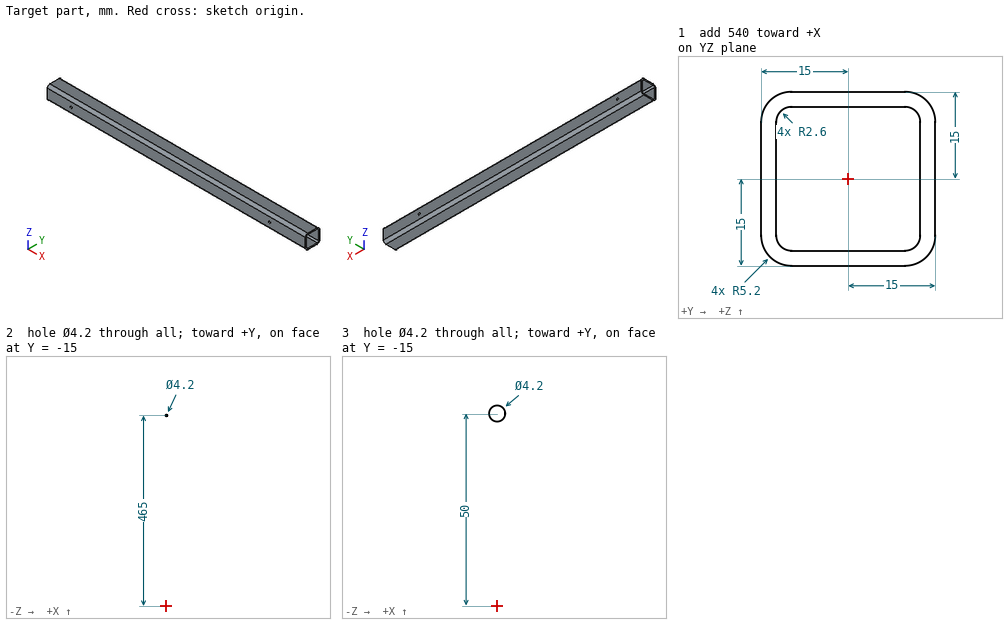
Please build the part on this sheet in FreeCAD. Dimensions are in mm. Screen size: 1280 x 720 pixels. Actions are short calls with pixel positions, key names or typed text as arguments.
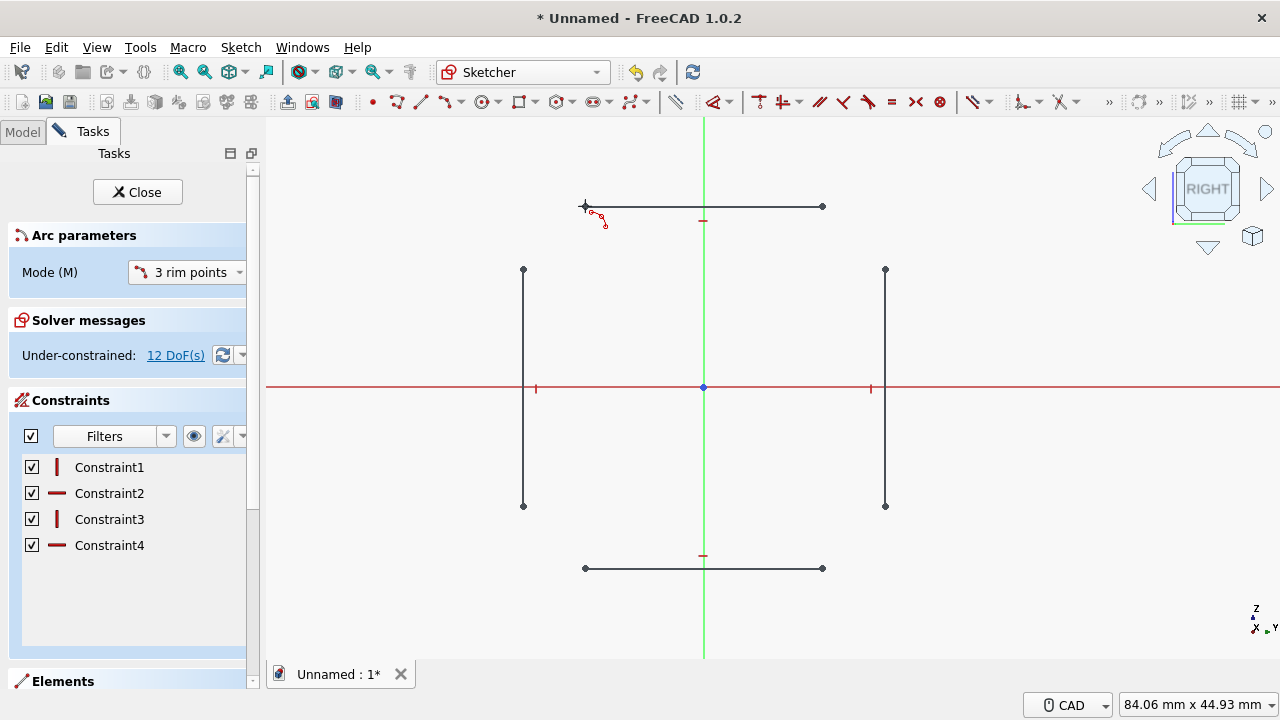
click(523, 507)
click(585, 569)
click(541, 550)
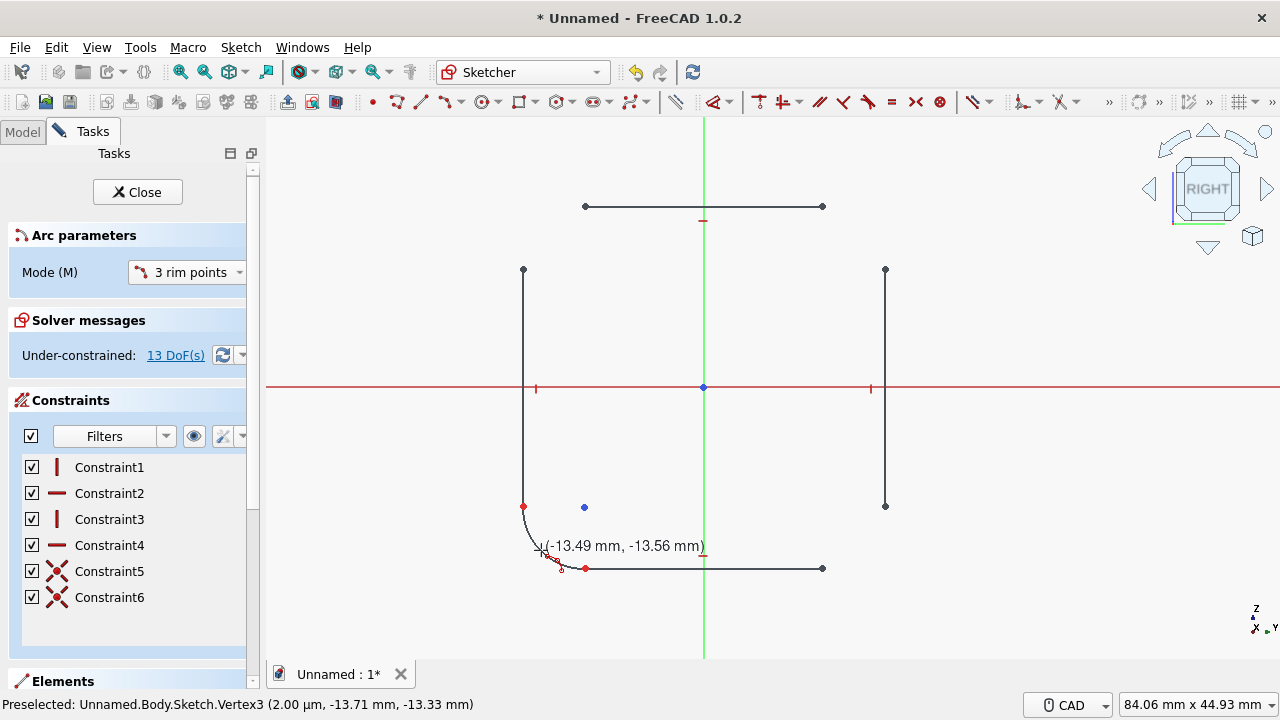
click(822, 569)
click(885, 507)
click(866, 550)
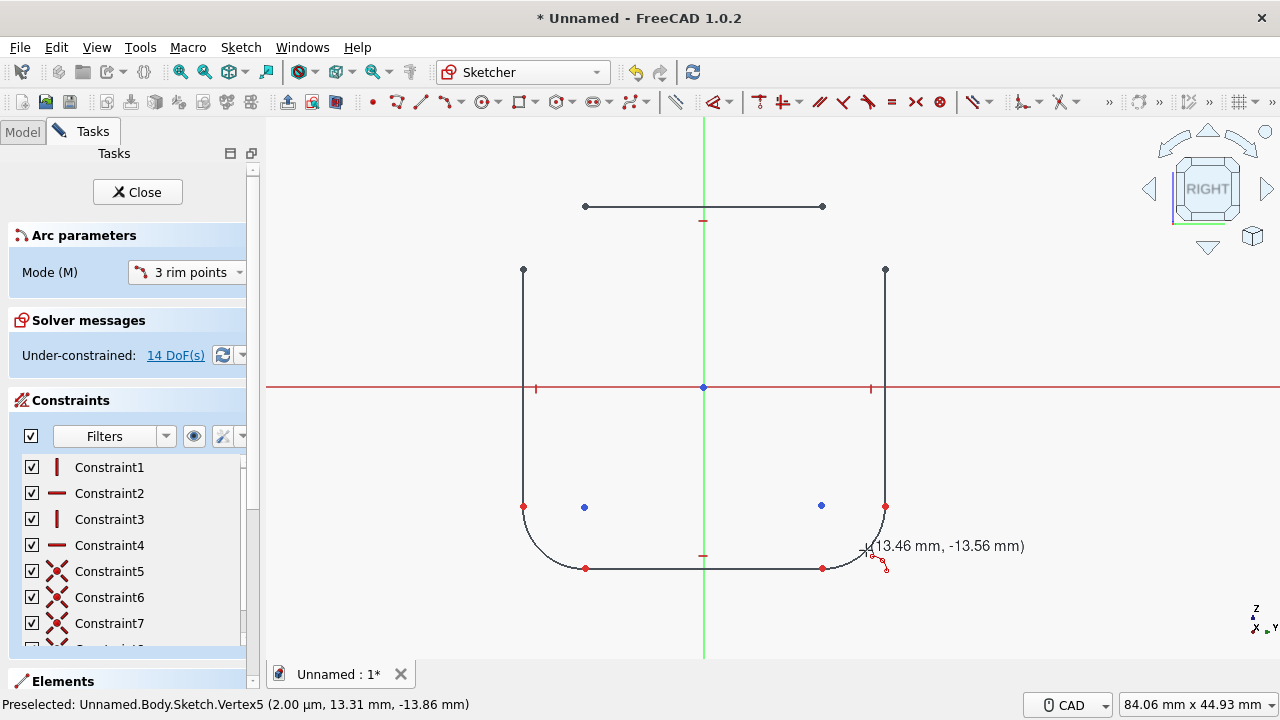
click(885, 270)
click(822, 207)
click(866, 225)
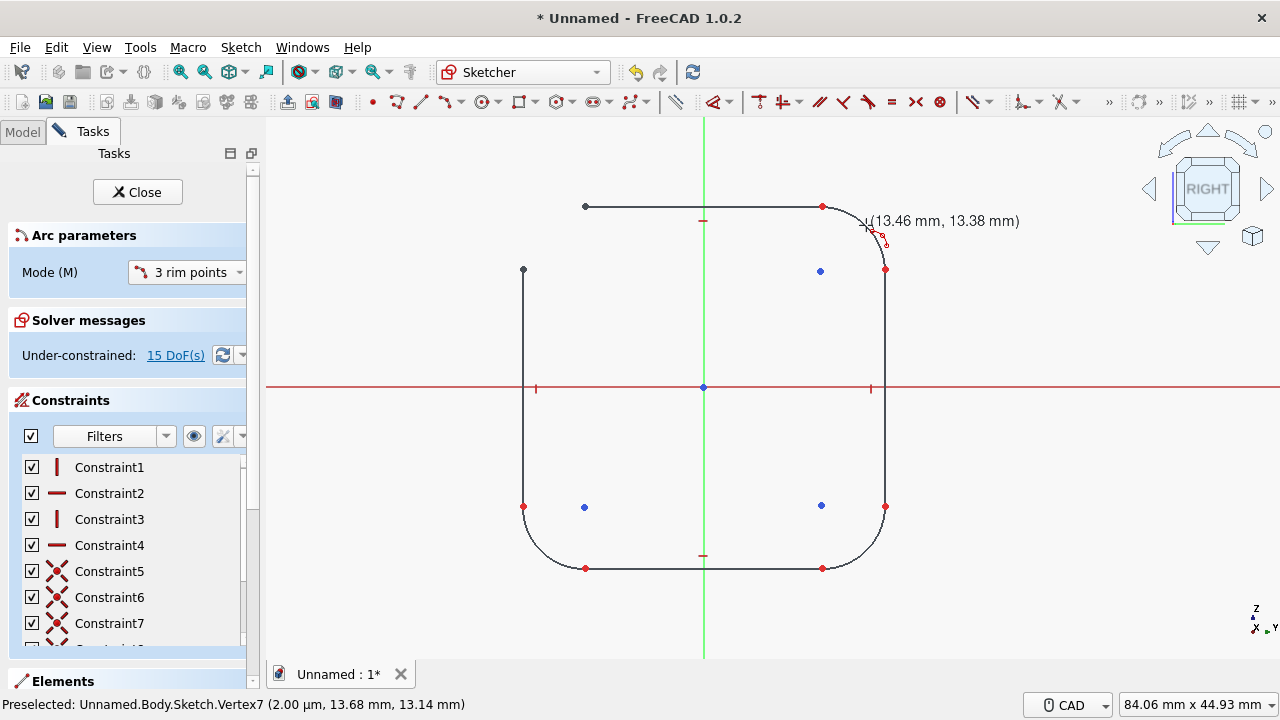
click(585, 207)
click(523, 270)
click(541, 225)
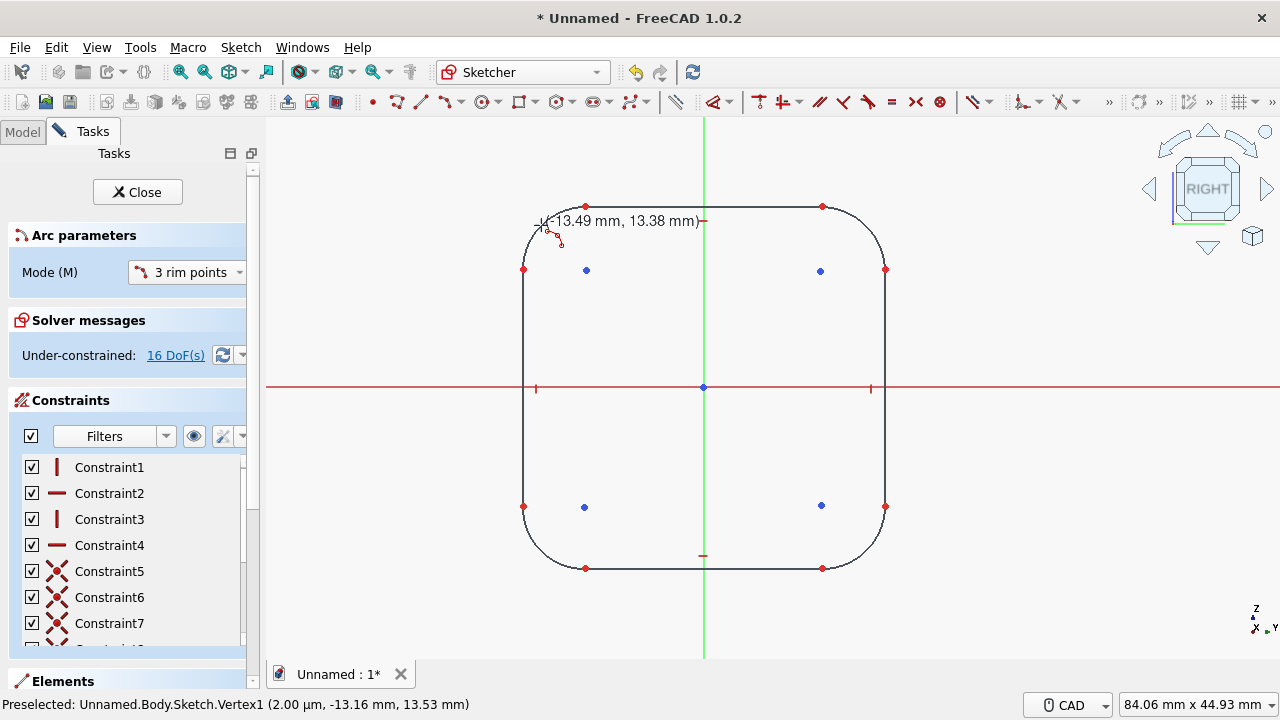
key(g)
key(l)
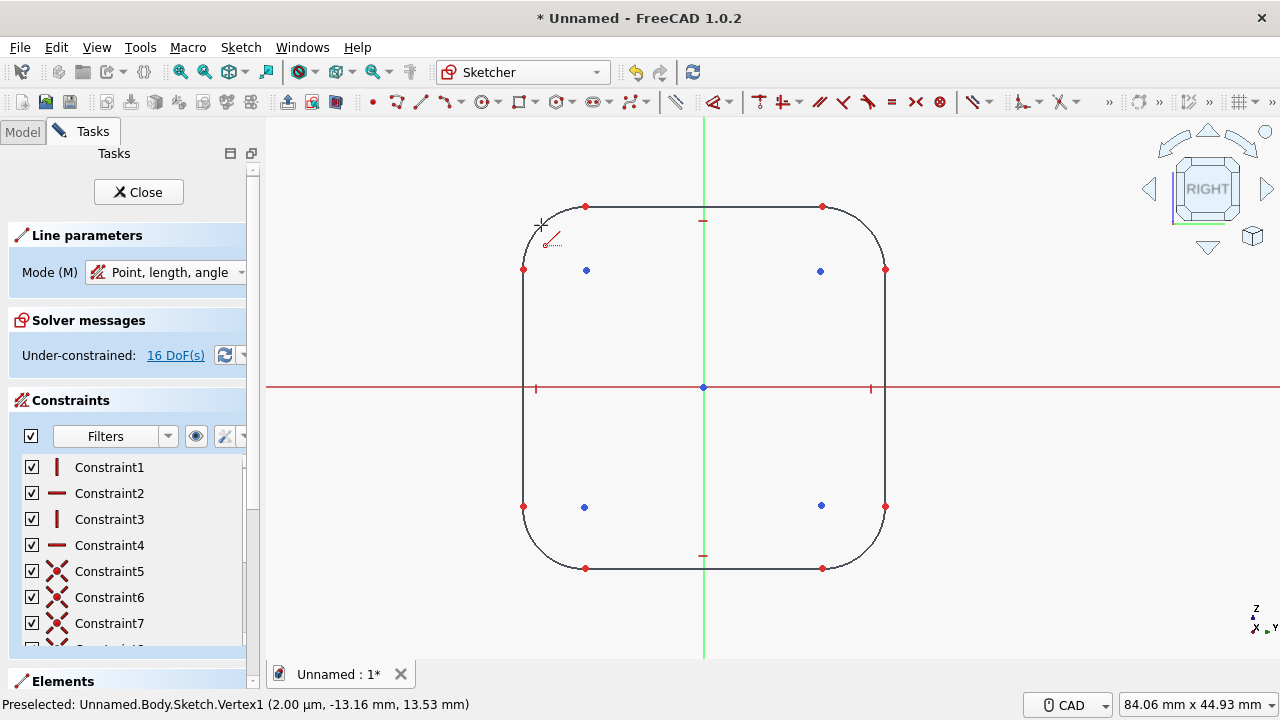
click(554, 506)
click(554, 269)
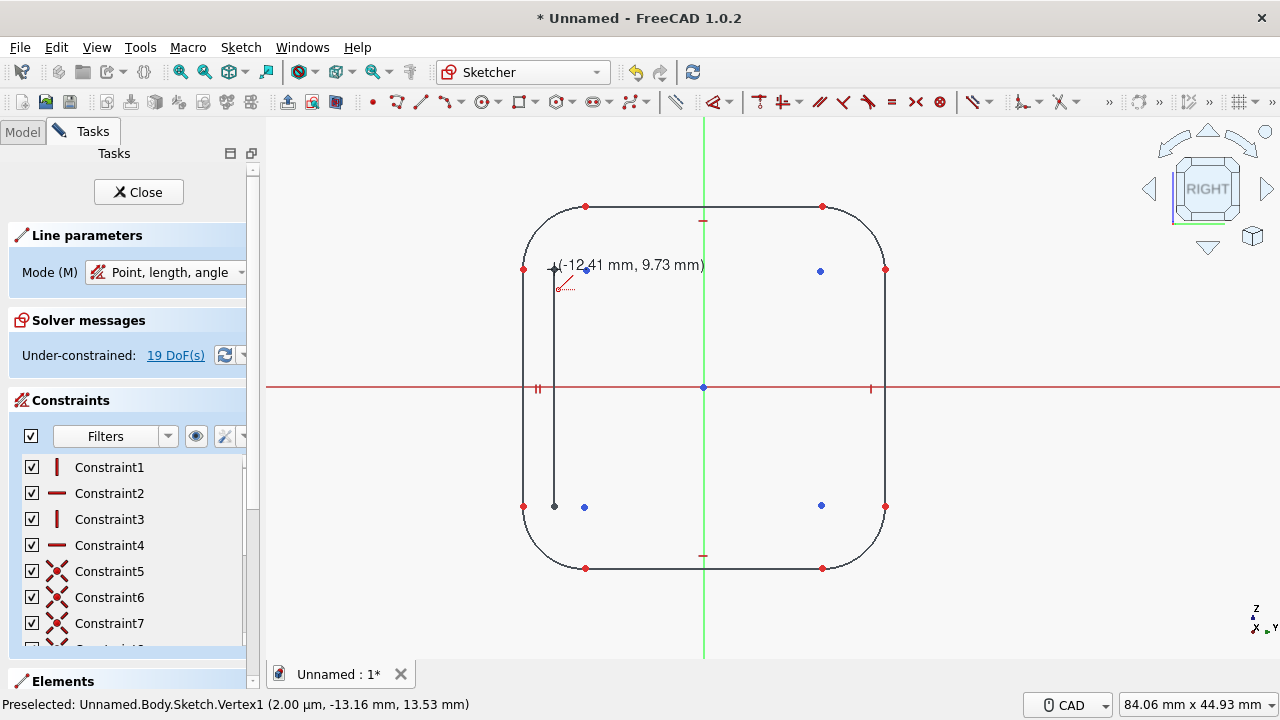
click(585, 238)
click(822, 238)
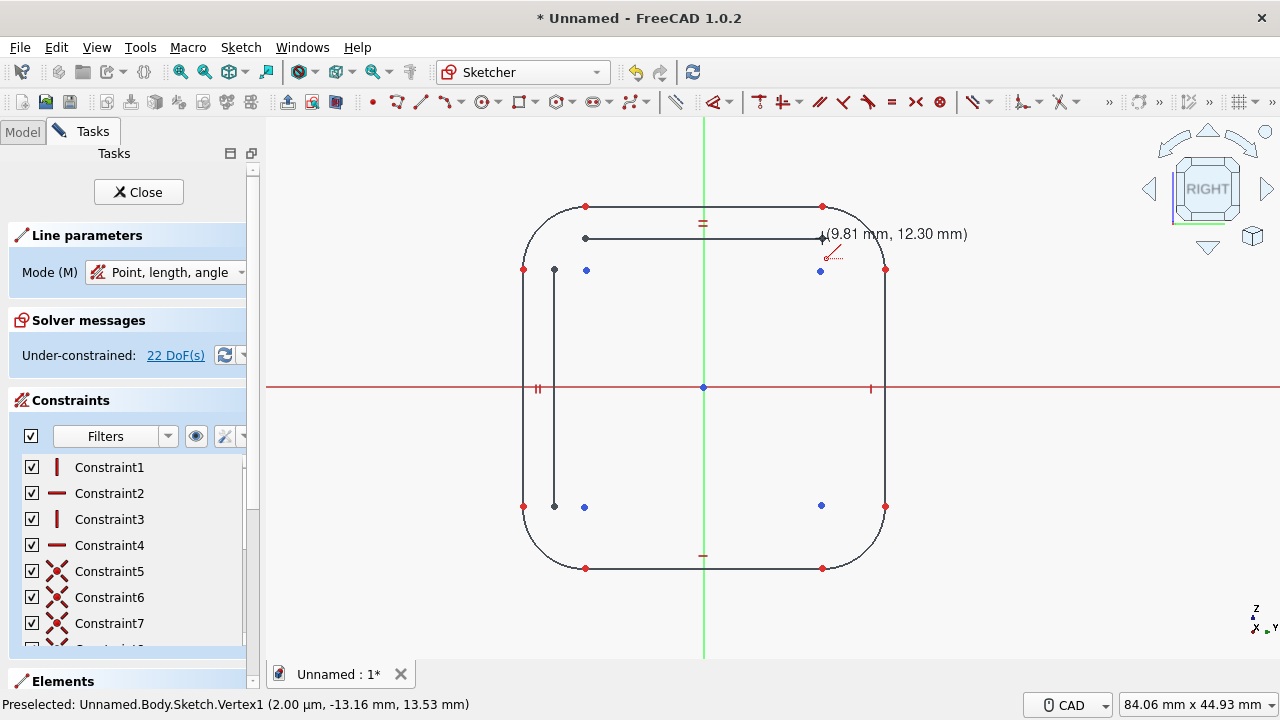
click(853, 269)
click(853, 506)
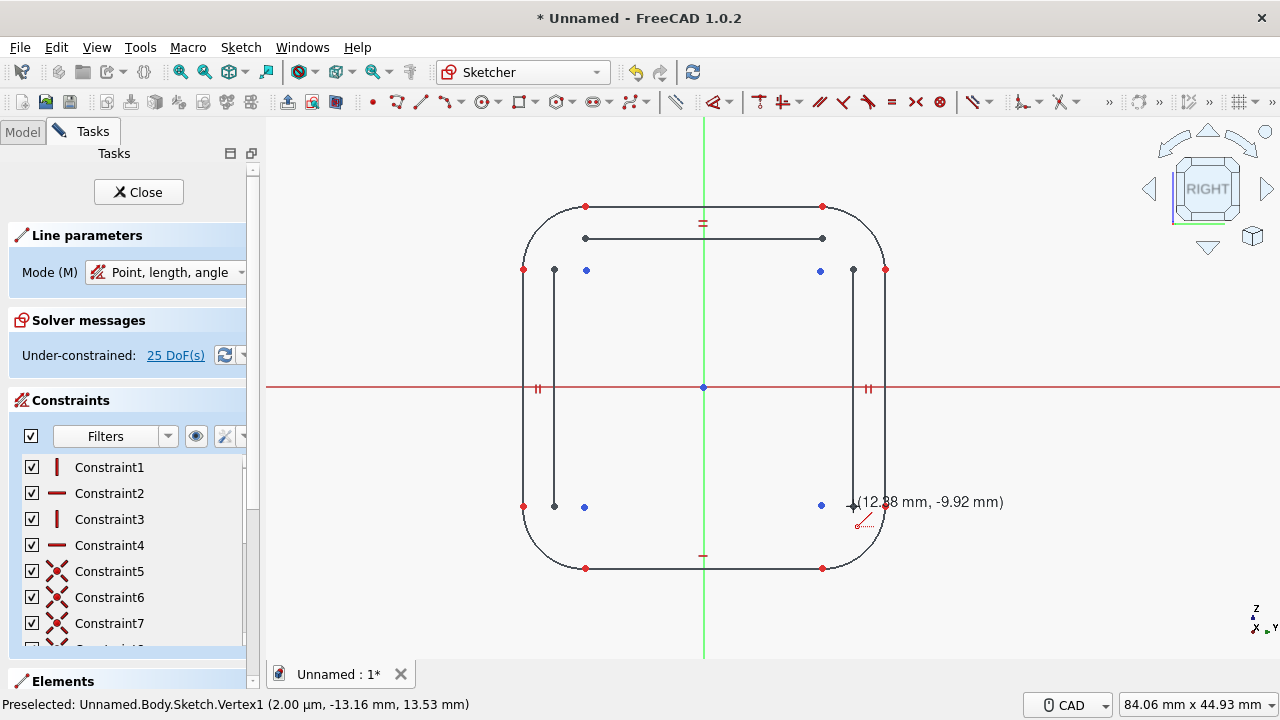
click(822, 537)
click(585, 537)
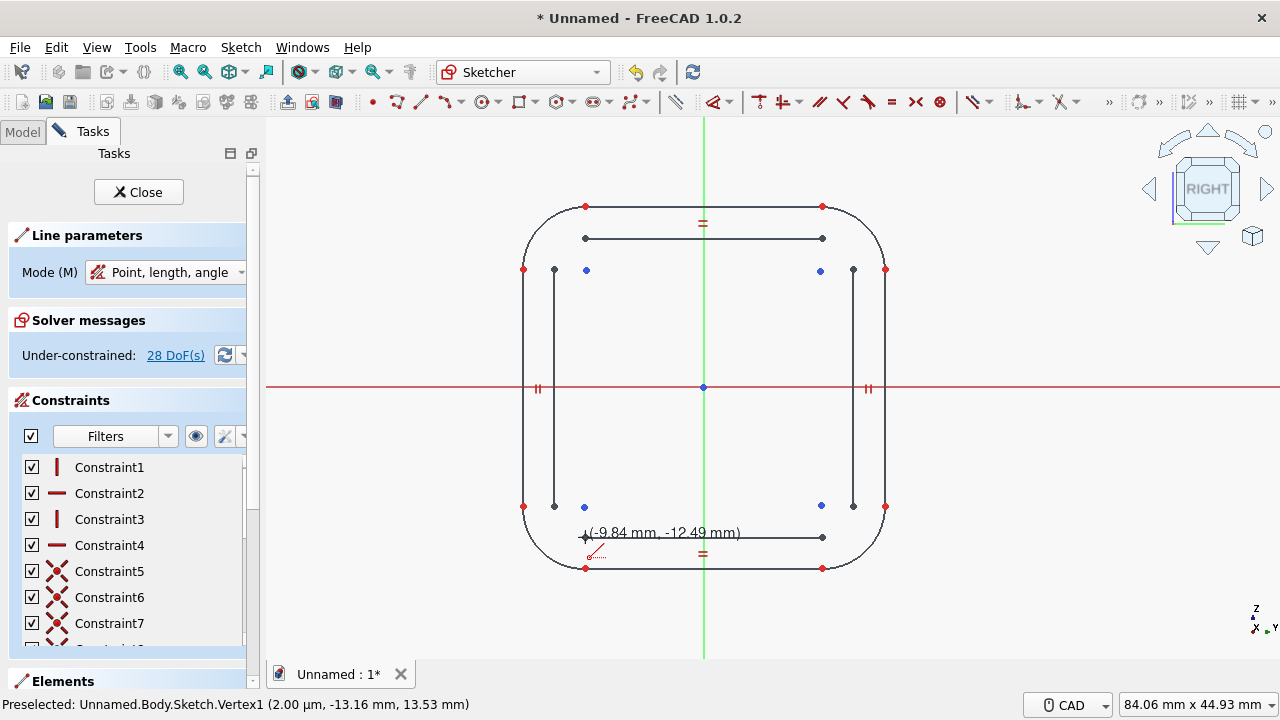
click(446, 102)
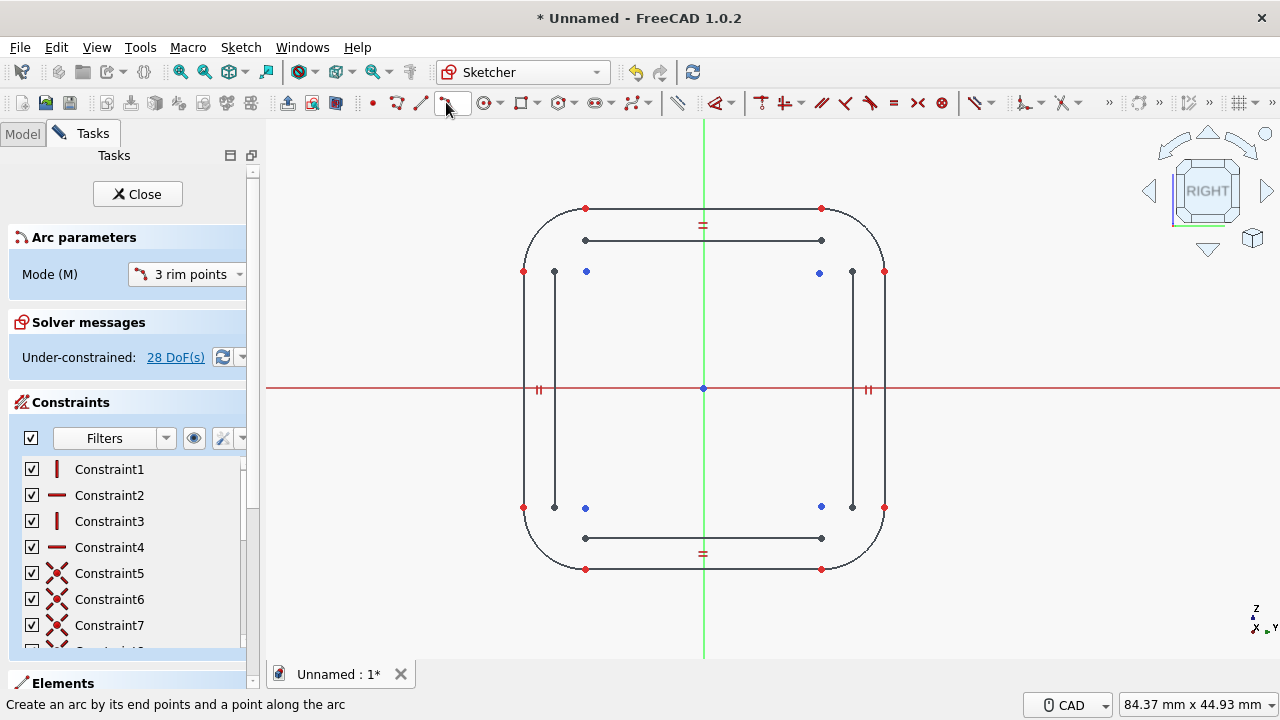
click(555, 271)
click(586, 241)